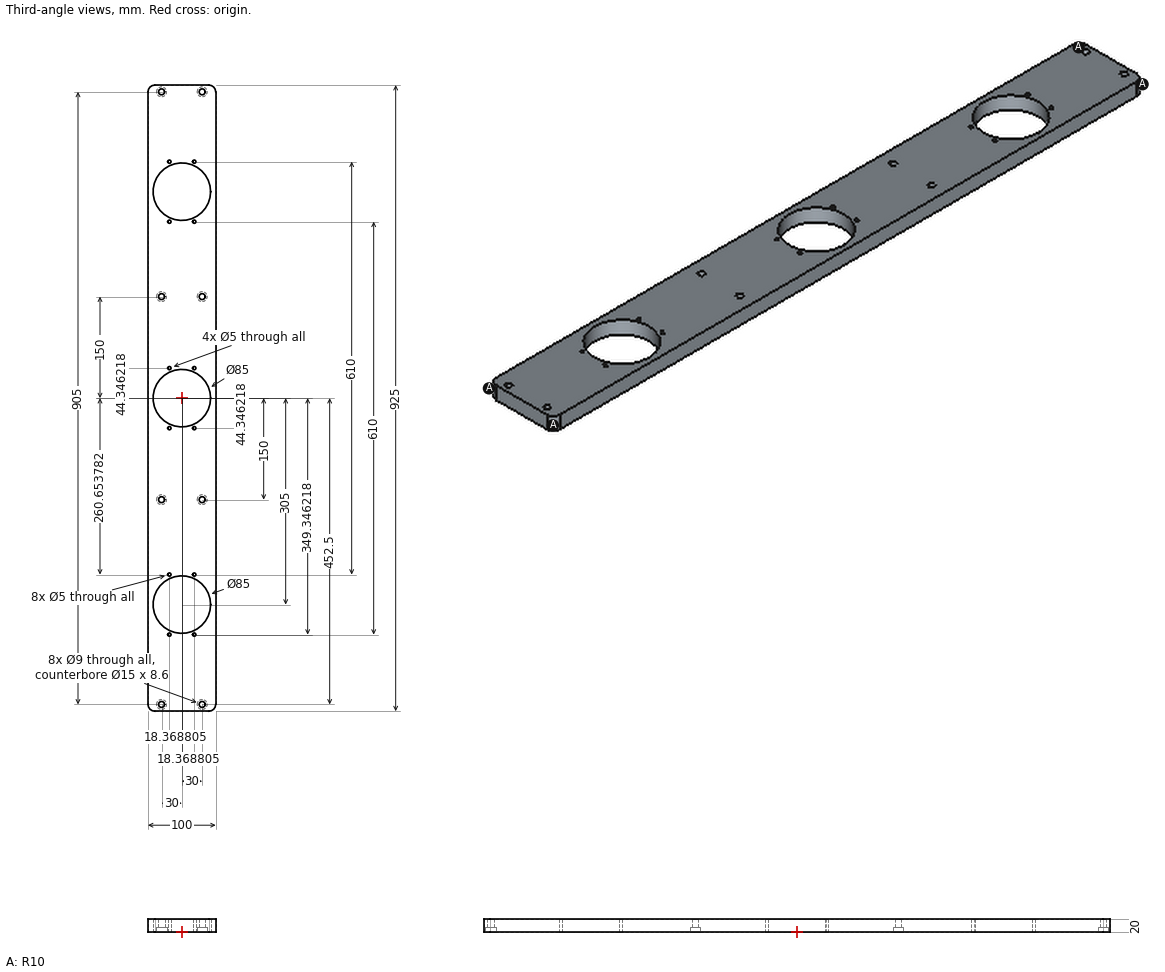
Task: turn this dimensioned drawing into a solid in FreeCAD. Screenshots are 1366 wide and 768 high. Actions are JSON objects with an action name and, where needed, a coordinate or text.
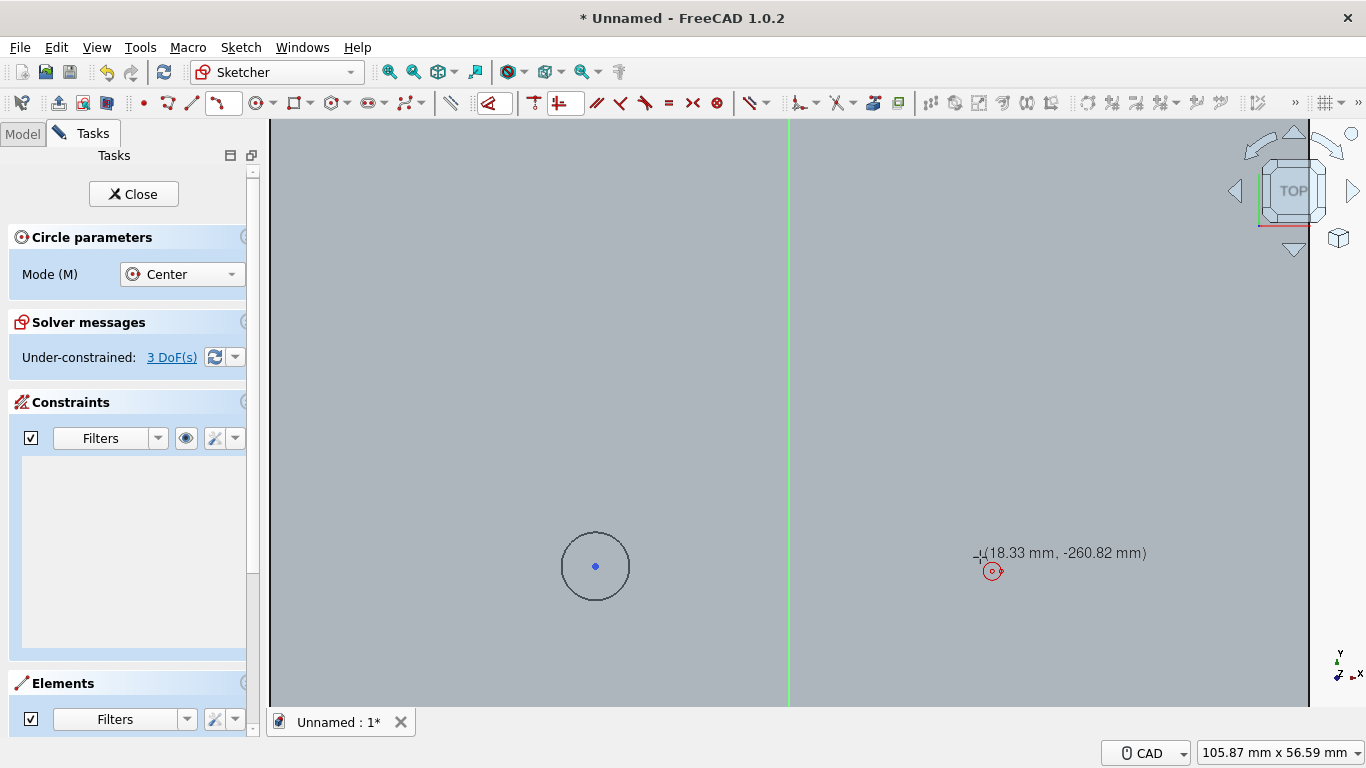
{"action": "scroll", "coordinate": [745, 547], "scroll_direction": "down", "scroll_amount": 15}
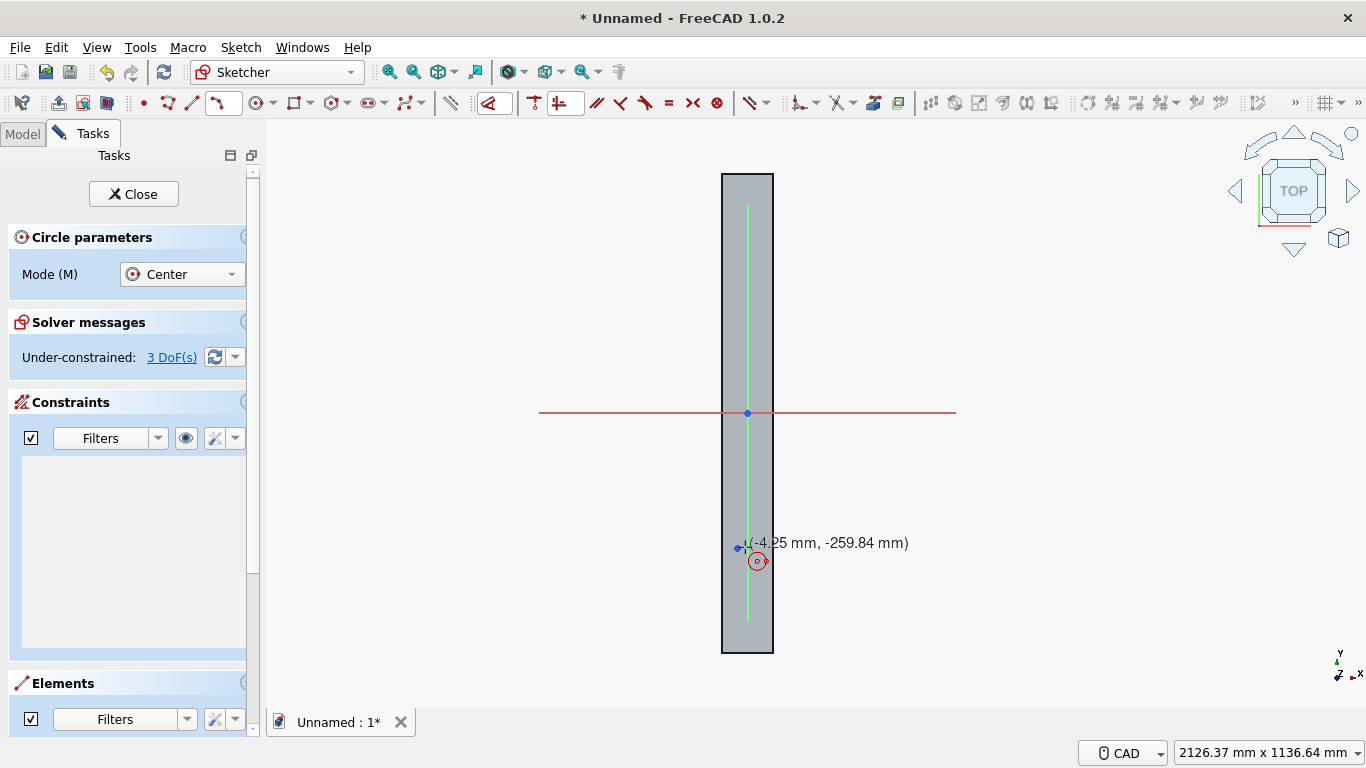
{"action": "scroll", "coordinate": [757, 548], "scroll_direction": "up", "scroll_amount": 3}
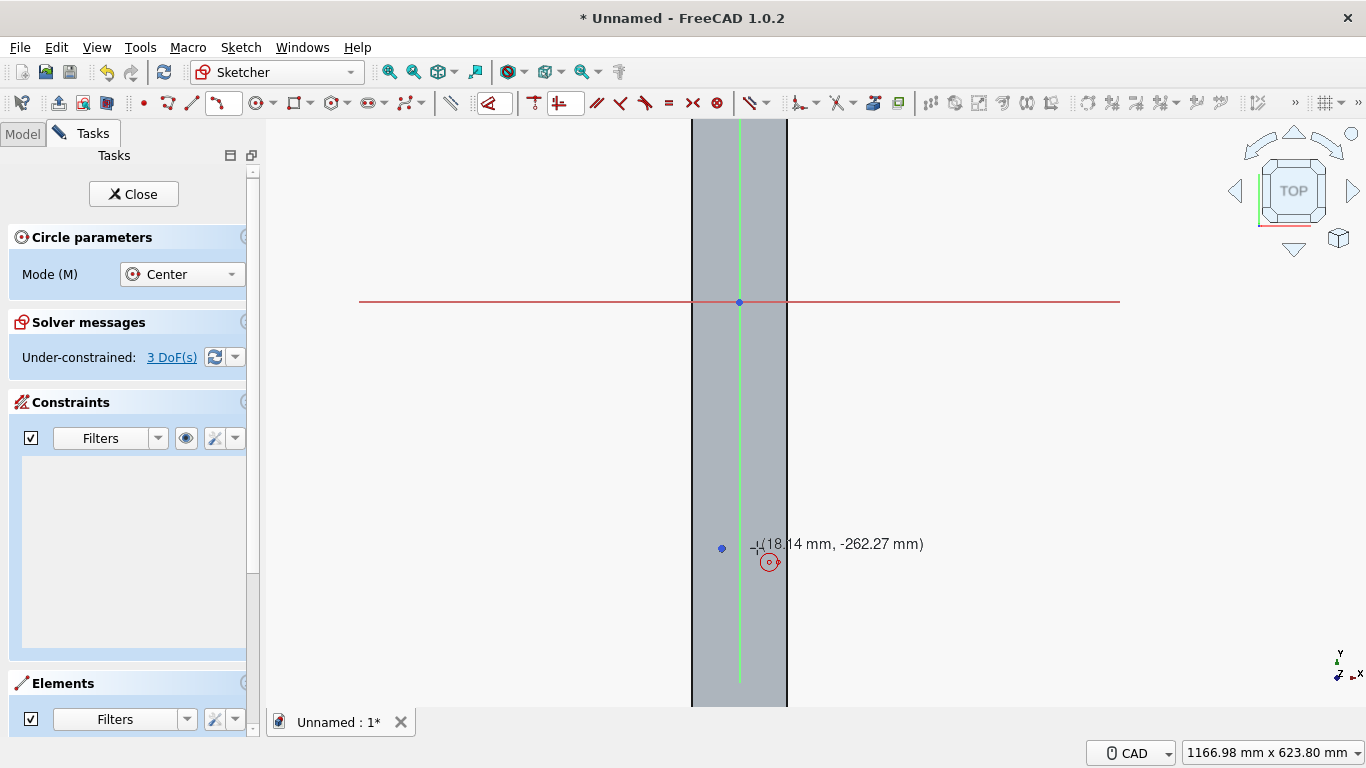
{"action": "left_click", "coordinate": [757, 548]}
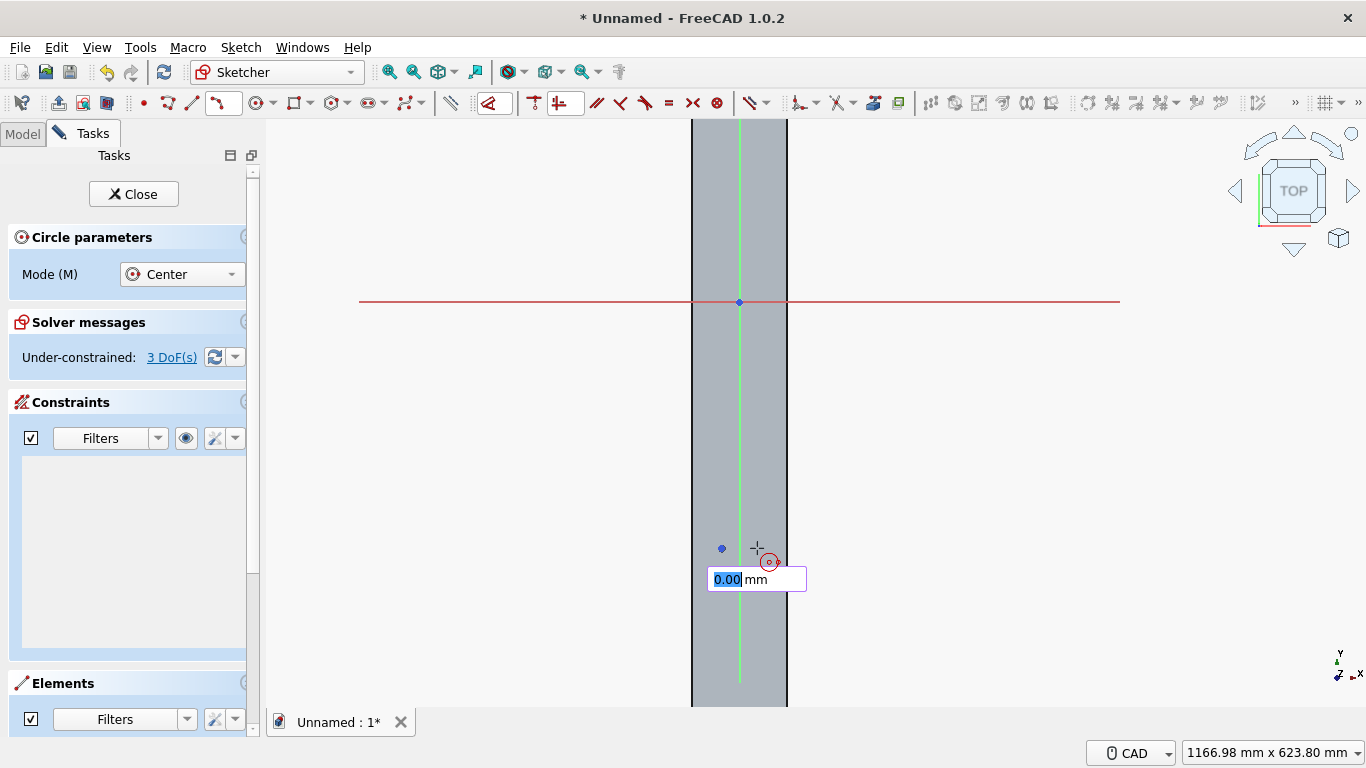
{"action": "scroll", "coordinate": [759, 546], "scroll_direction": "up", "scroll_amount": 10}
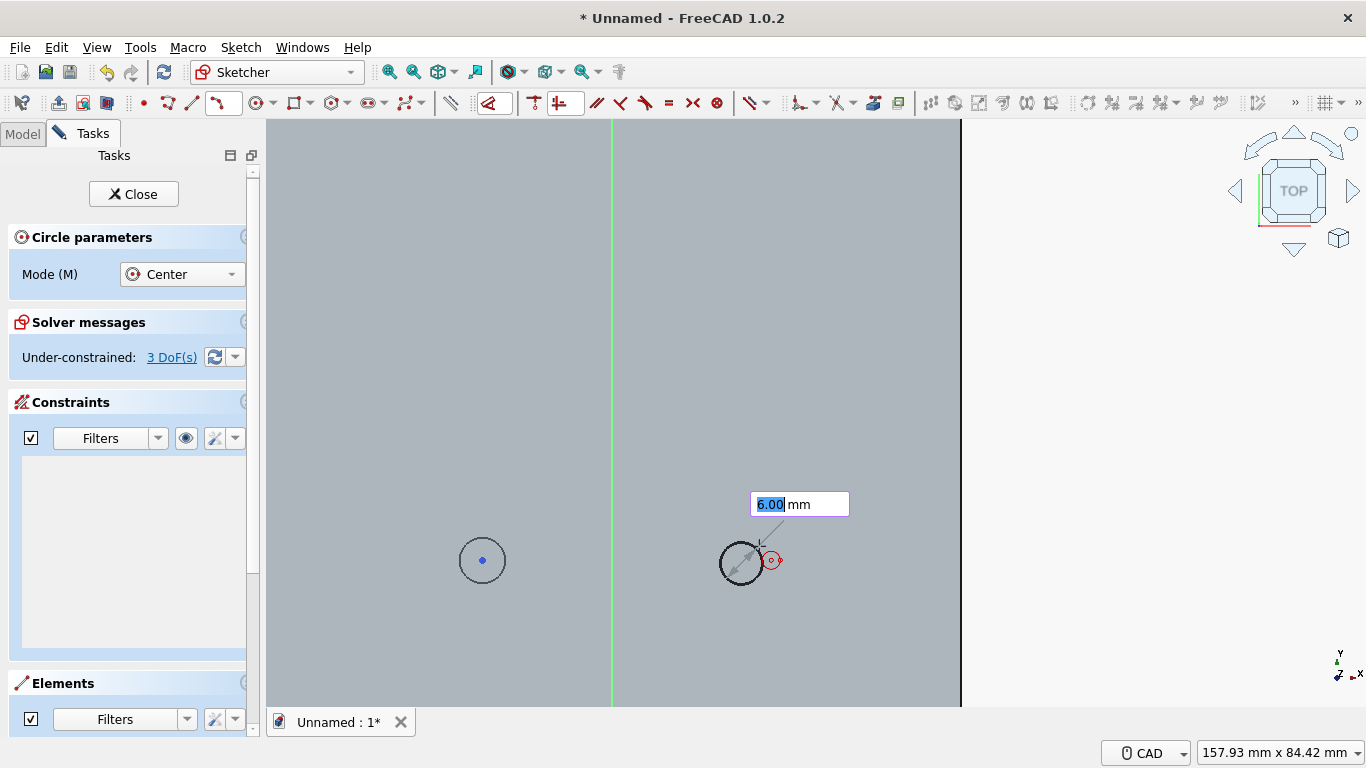
{"action": "left_click", "coordinate": [753, 542]}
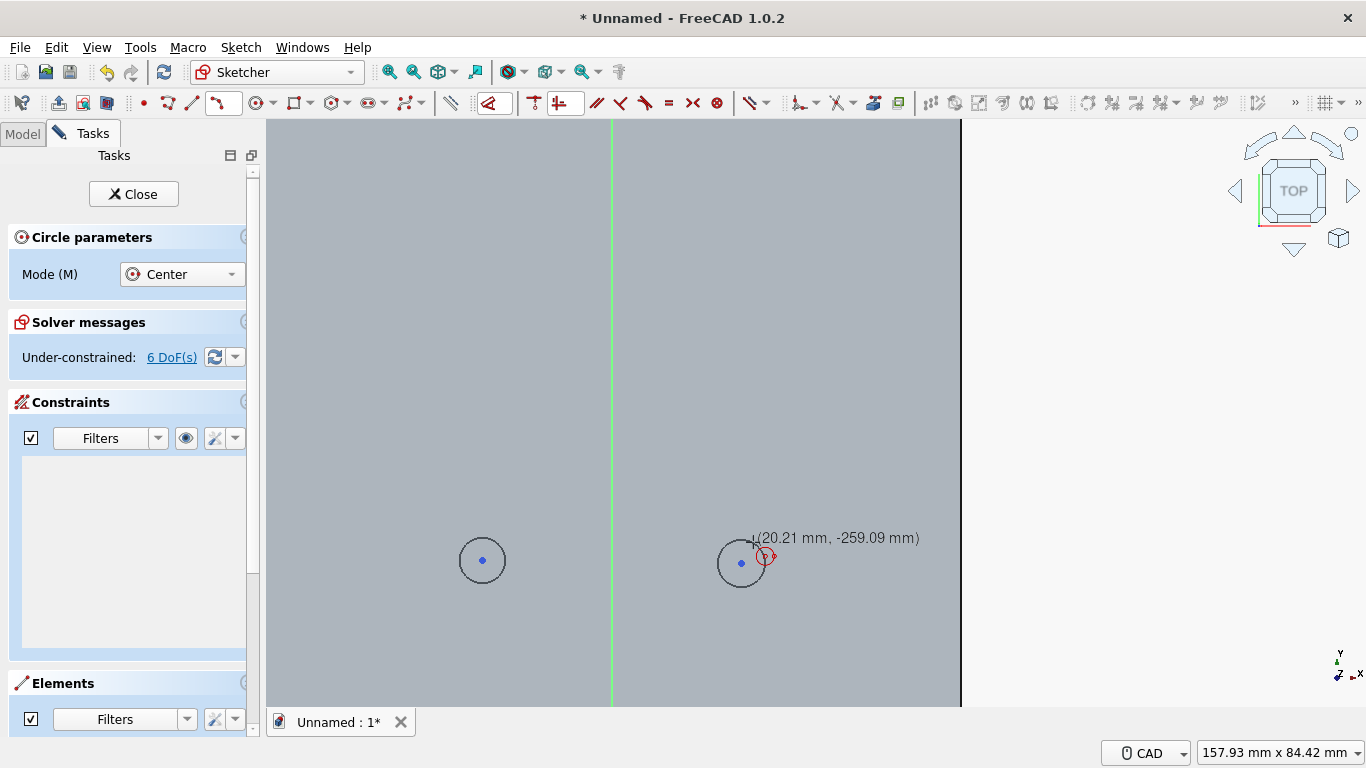
{"action": "scroll", "coordinate": [758, 547], "scroll_direction": "down", "scroll_amount": 13}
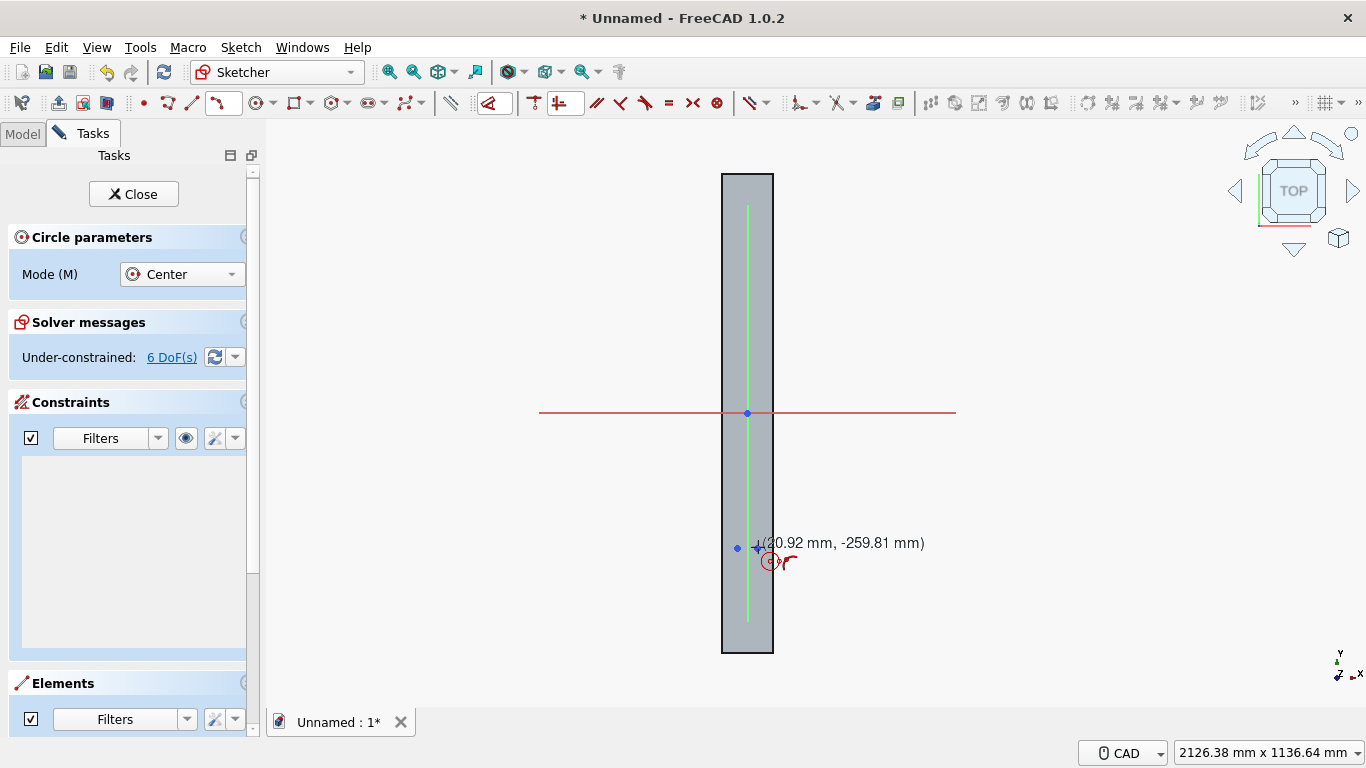
{"action": "scroll", "coordinate": [757, 594], "scroll_direction": "up", "scroll_amount": 15}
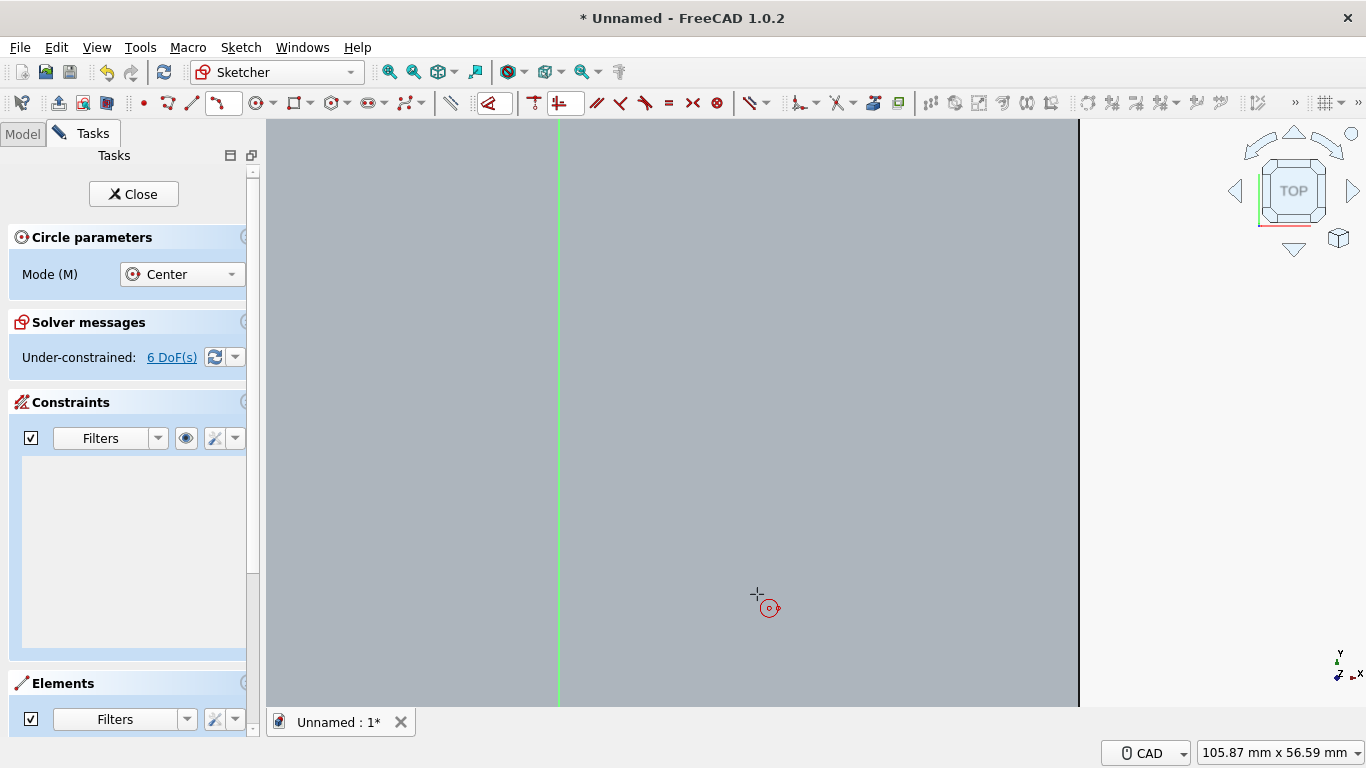
{"action": "scroll", "coordinate": [757, 594], "scroll_direction": "down", "scroll_amount": 15}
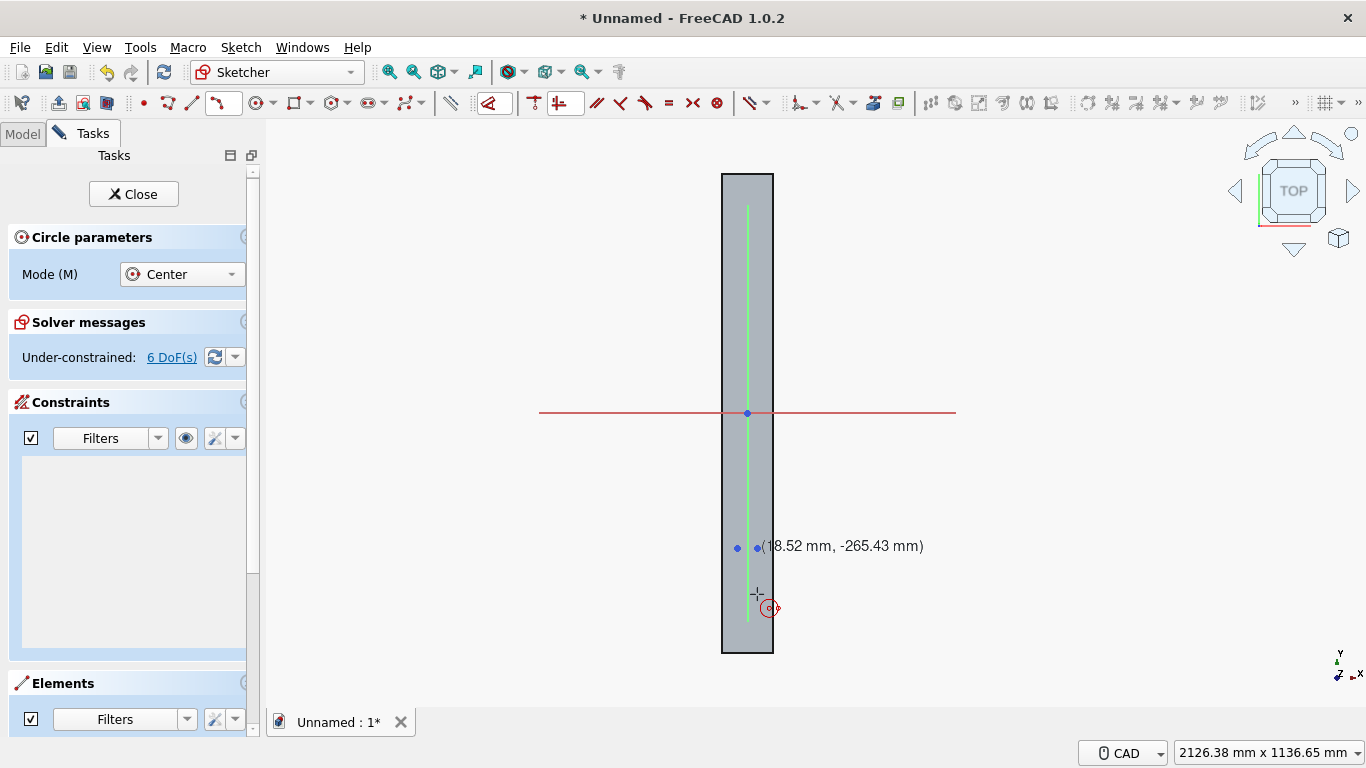
{"action": "scroll", "coordinate": [757, 594], "scroll_direction": "up", "scroll_amount": 3}